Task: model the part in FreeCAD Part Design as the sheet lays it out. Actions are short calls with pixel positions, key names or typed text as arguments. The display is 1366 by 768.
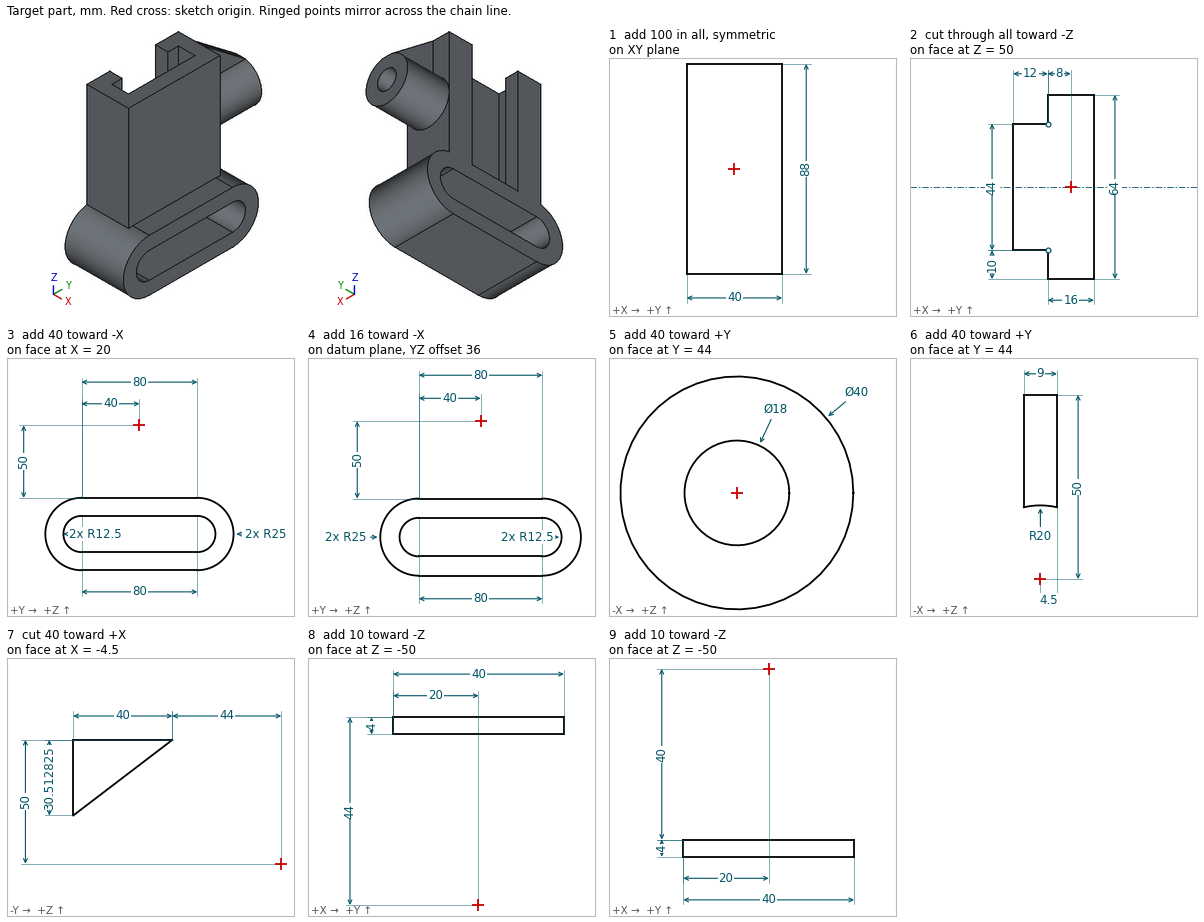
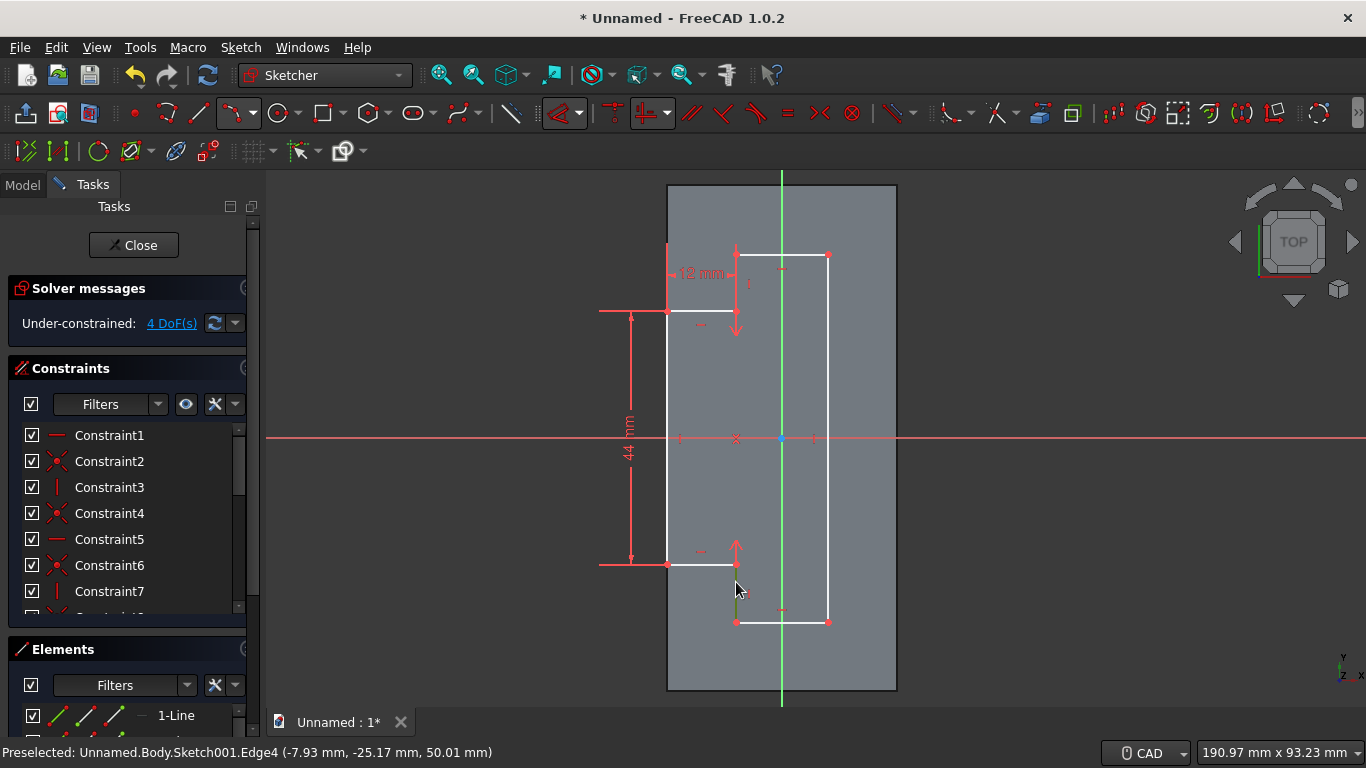
key(i)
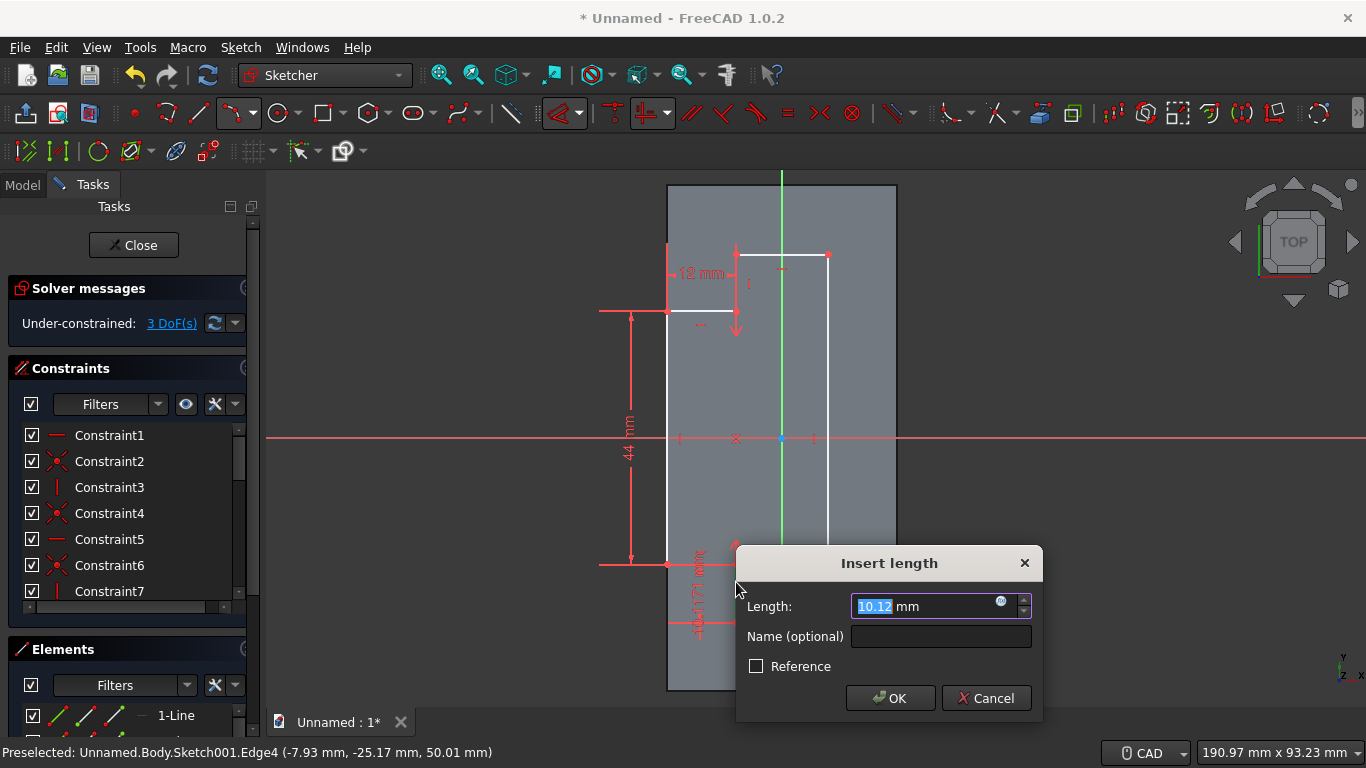
text(10)
key(Return)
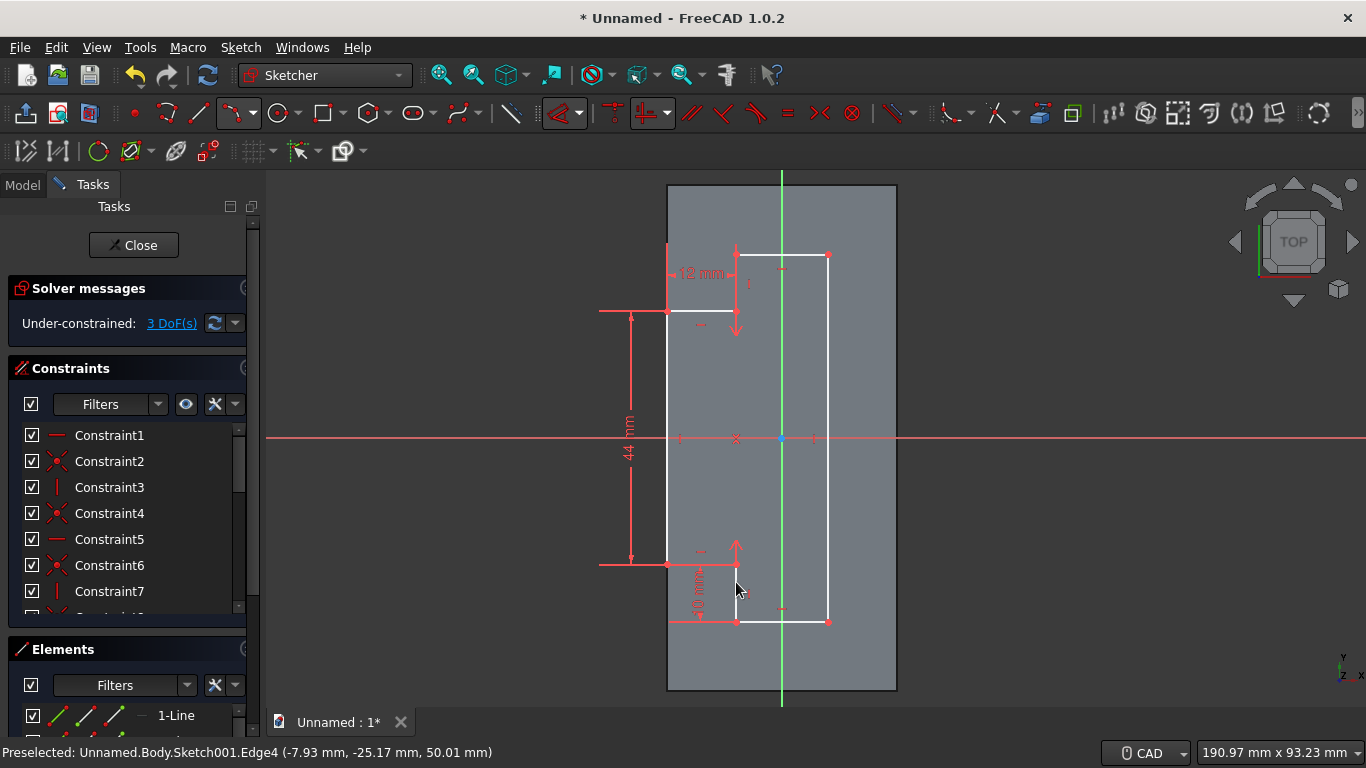
click(764, 622)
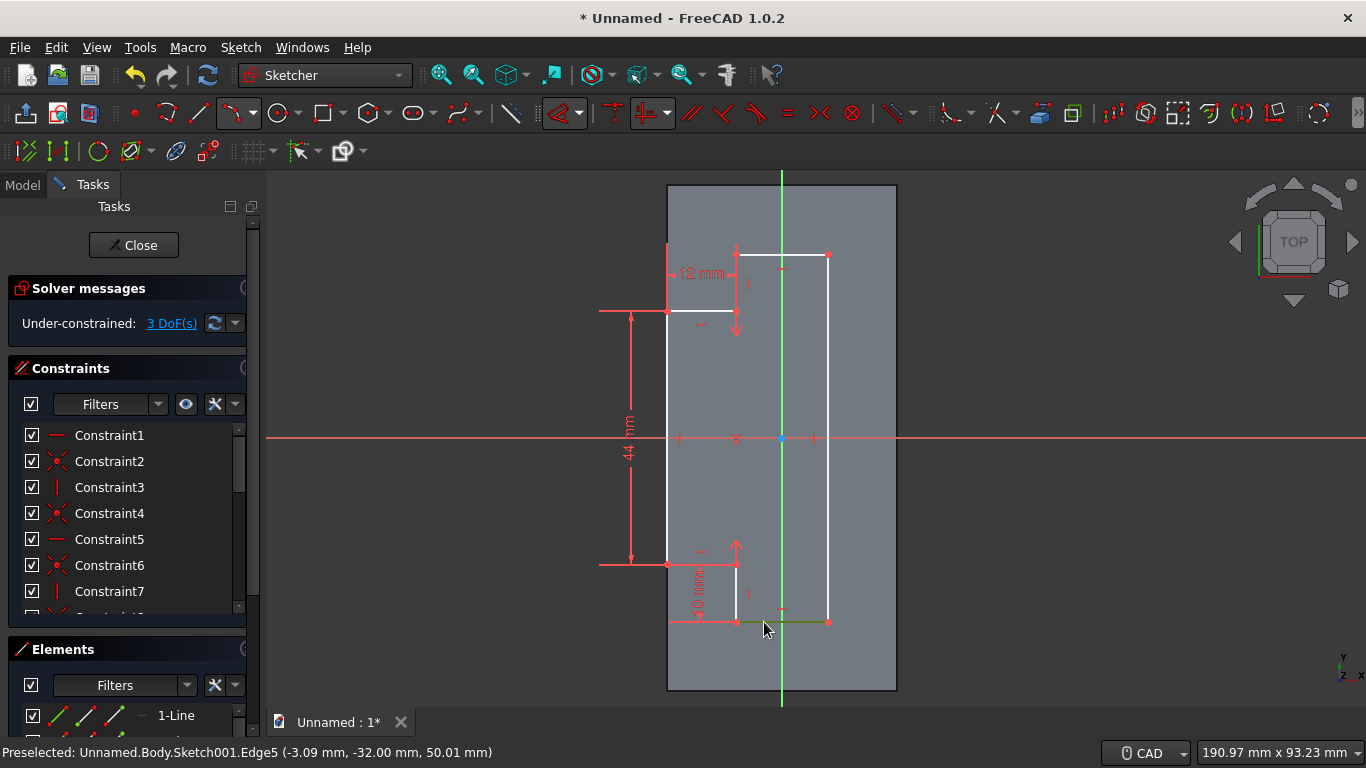
key(l)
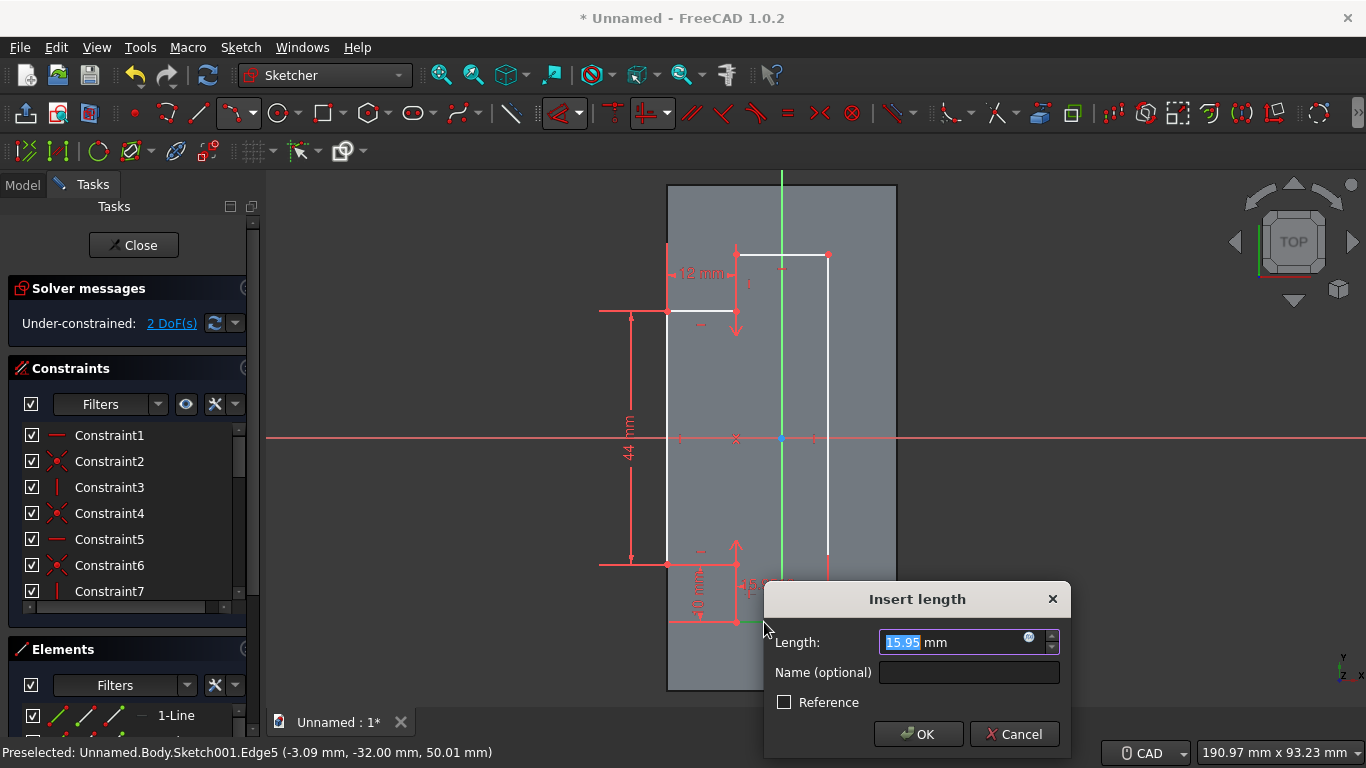
text(16)
key(Return)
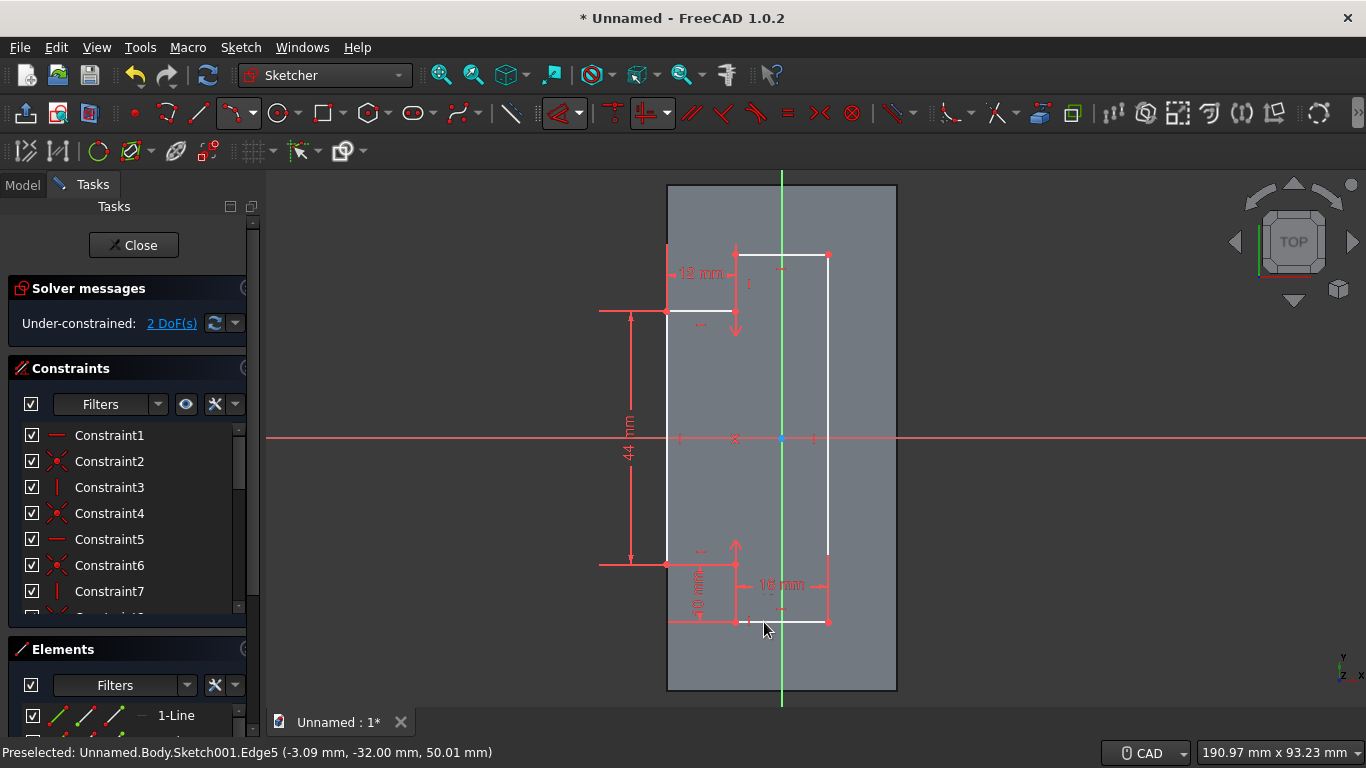
click(828, 512)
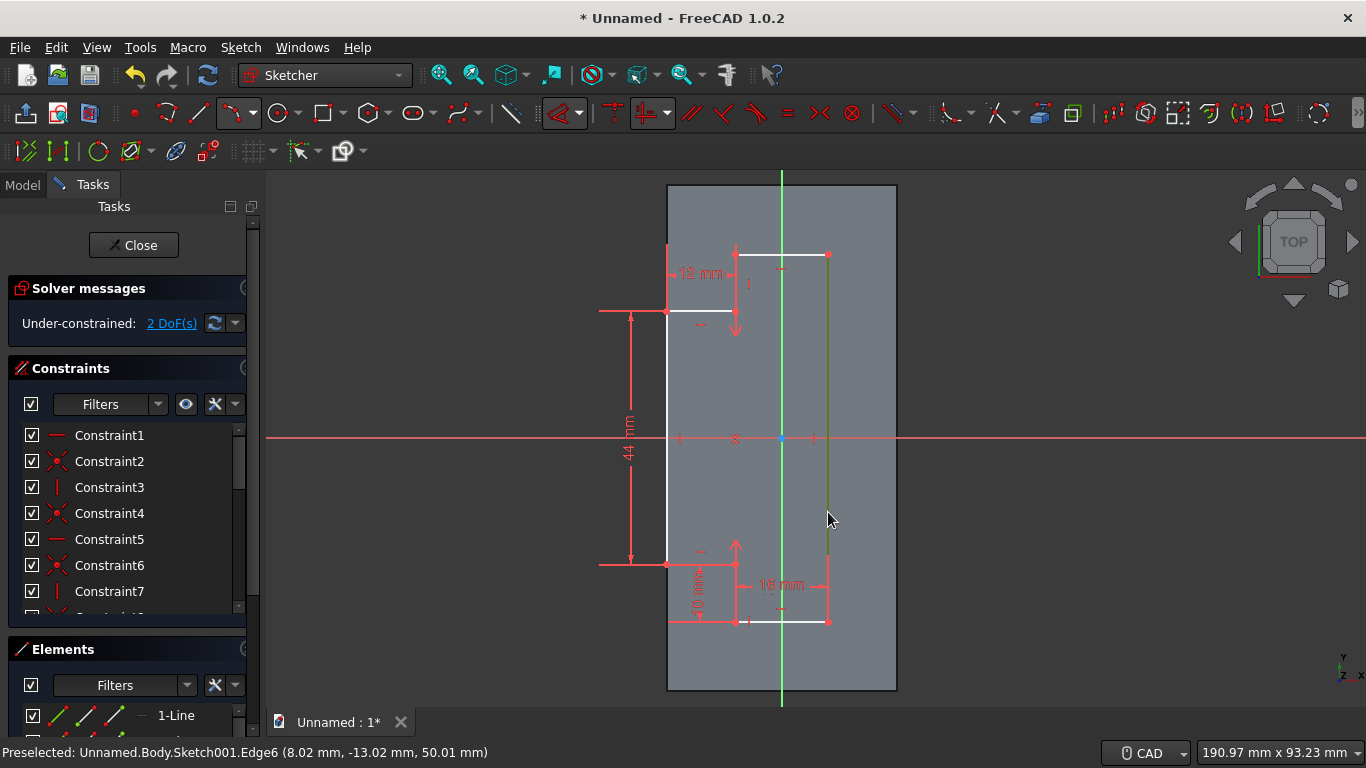
click(582, 114)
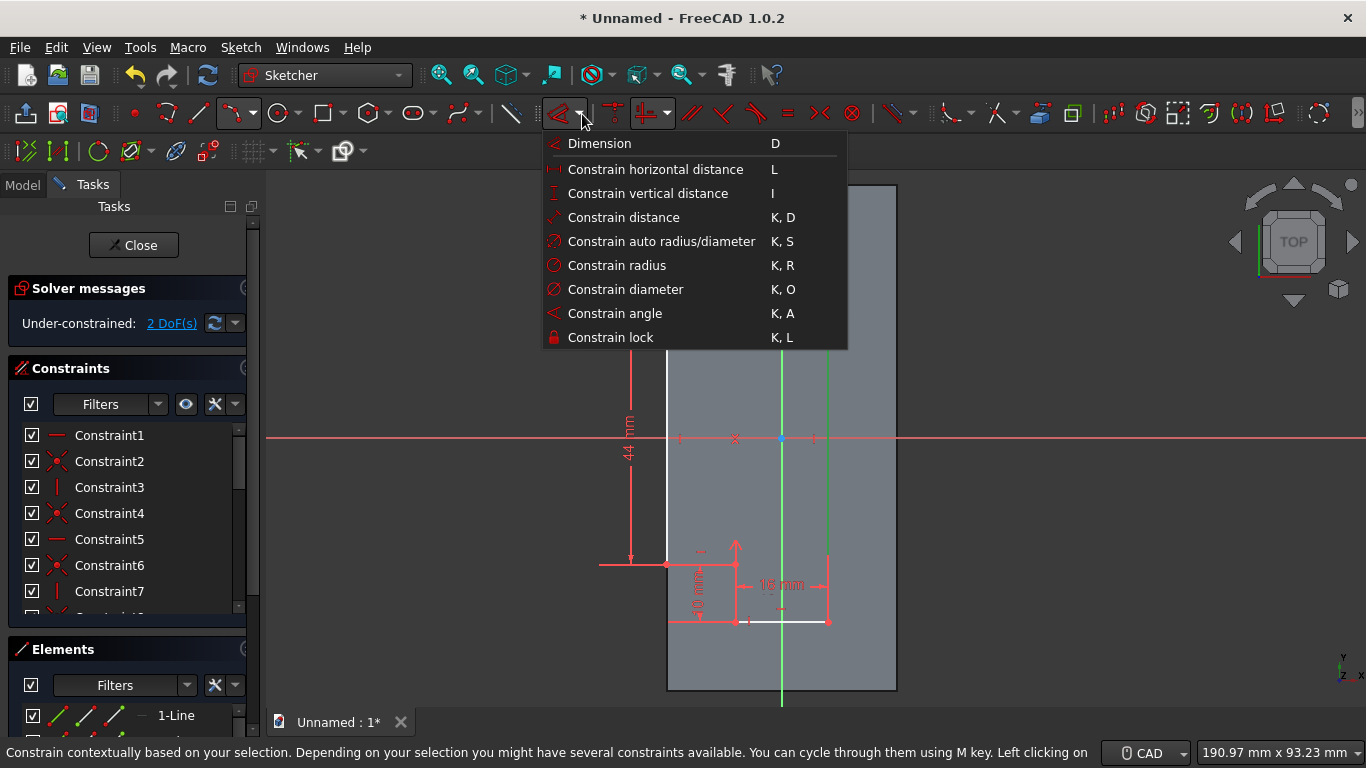
click(695, 193)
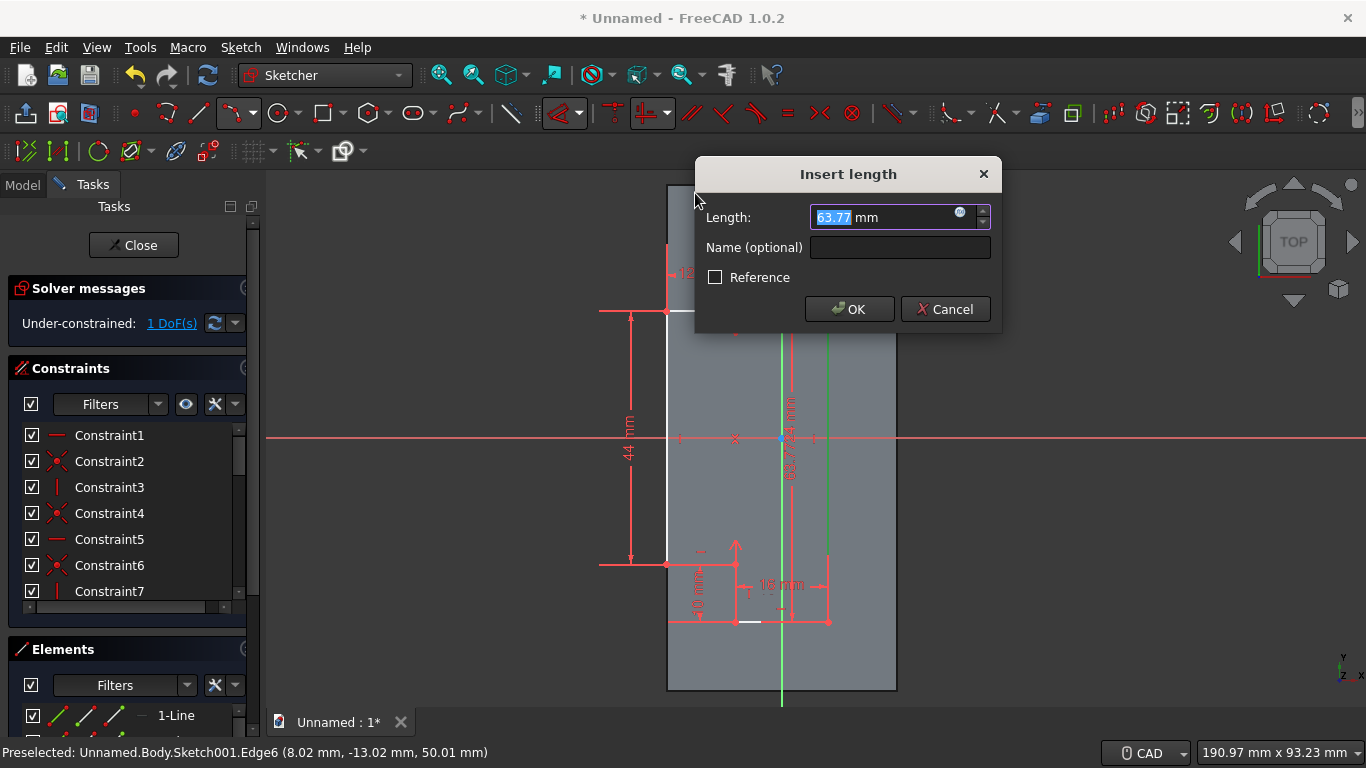
text(64)
key(Return)